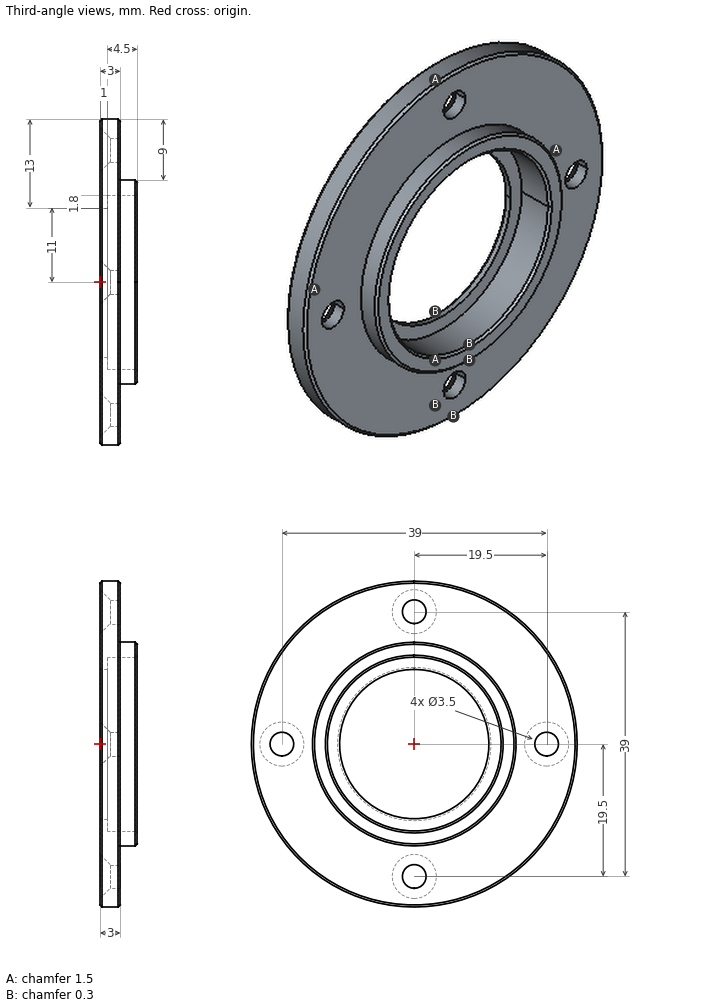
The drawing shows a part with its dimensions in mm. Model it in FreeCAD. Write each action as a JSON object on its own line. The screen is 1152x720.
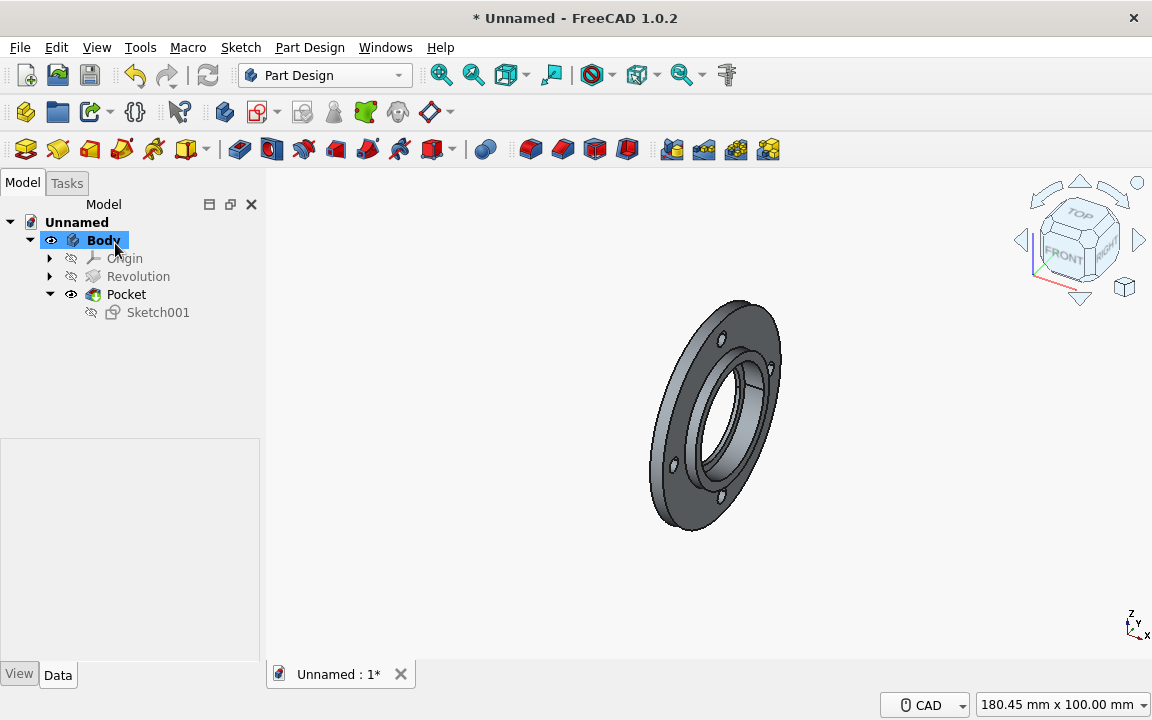
{"action": "key", "text": "0"}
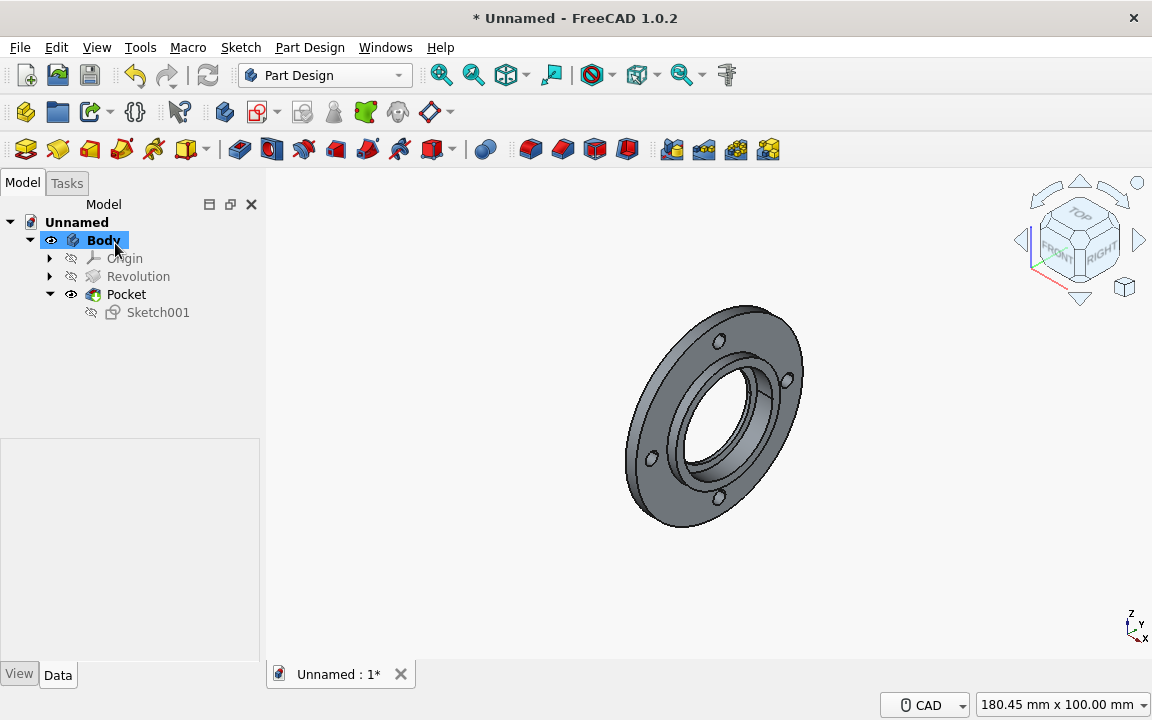
{"action": "key", "text": "2"}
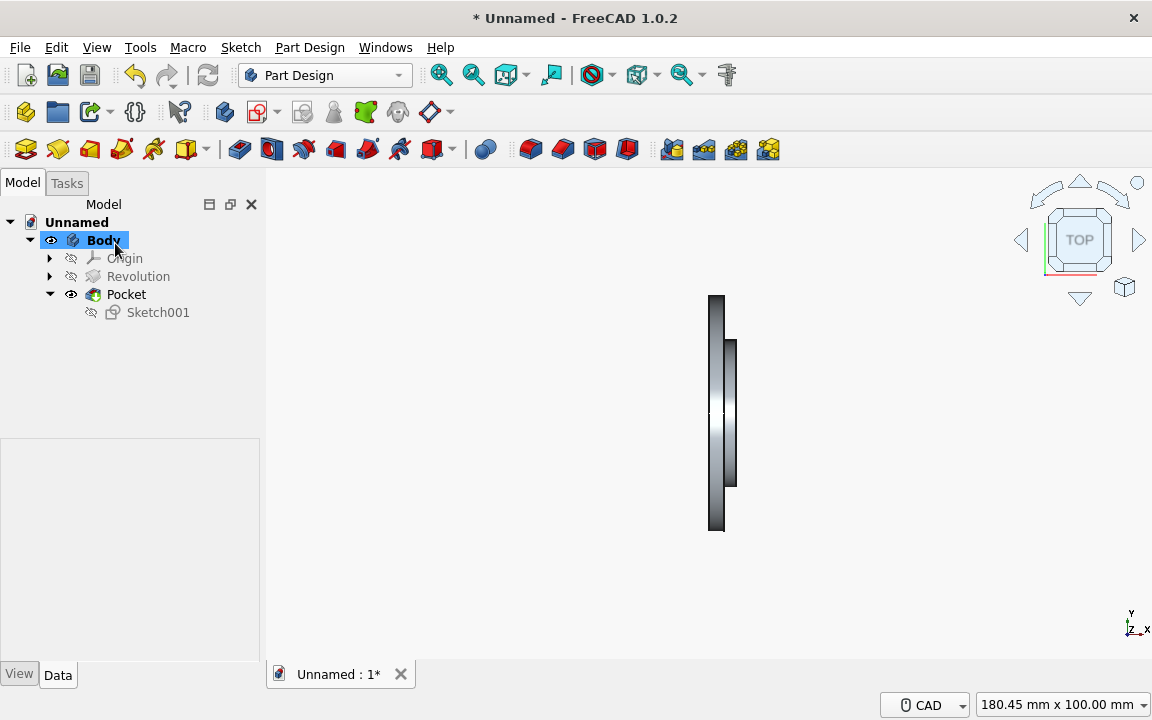
{"action": "key", "text": "1"}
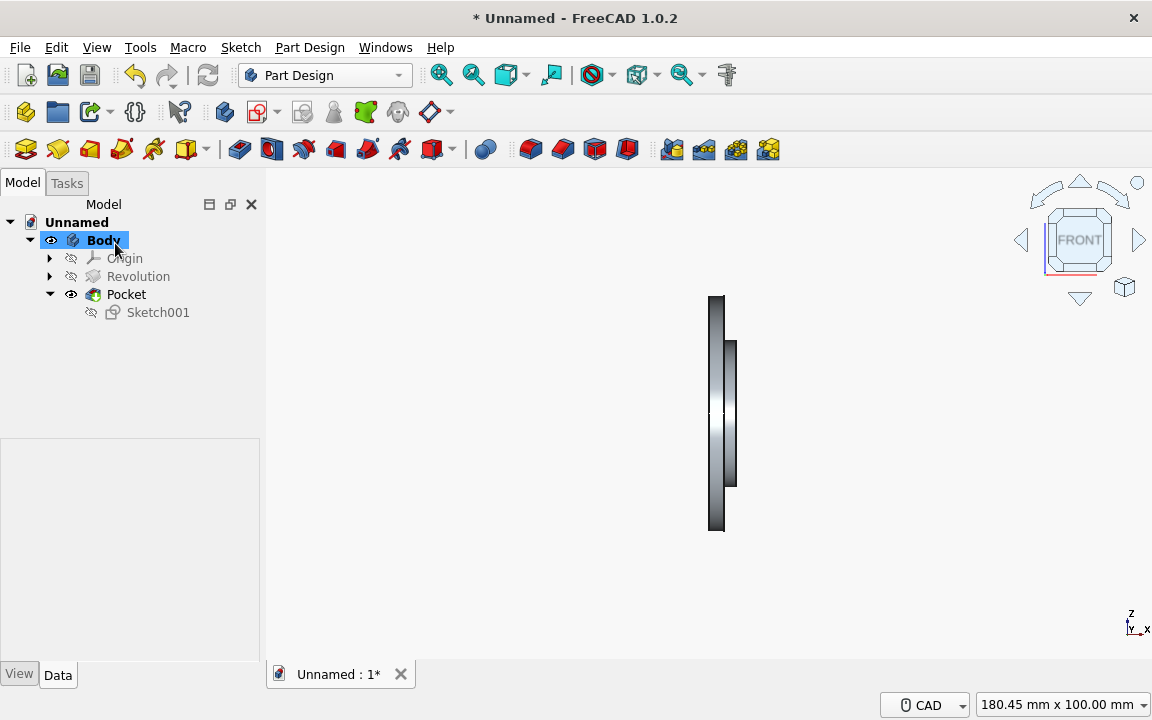
{"action": "key", "text": "3"}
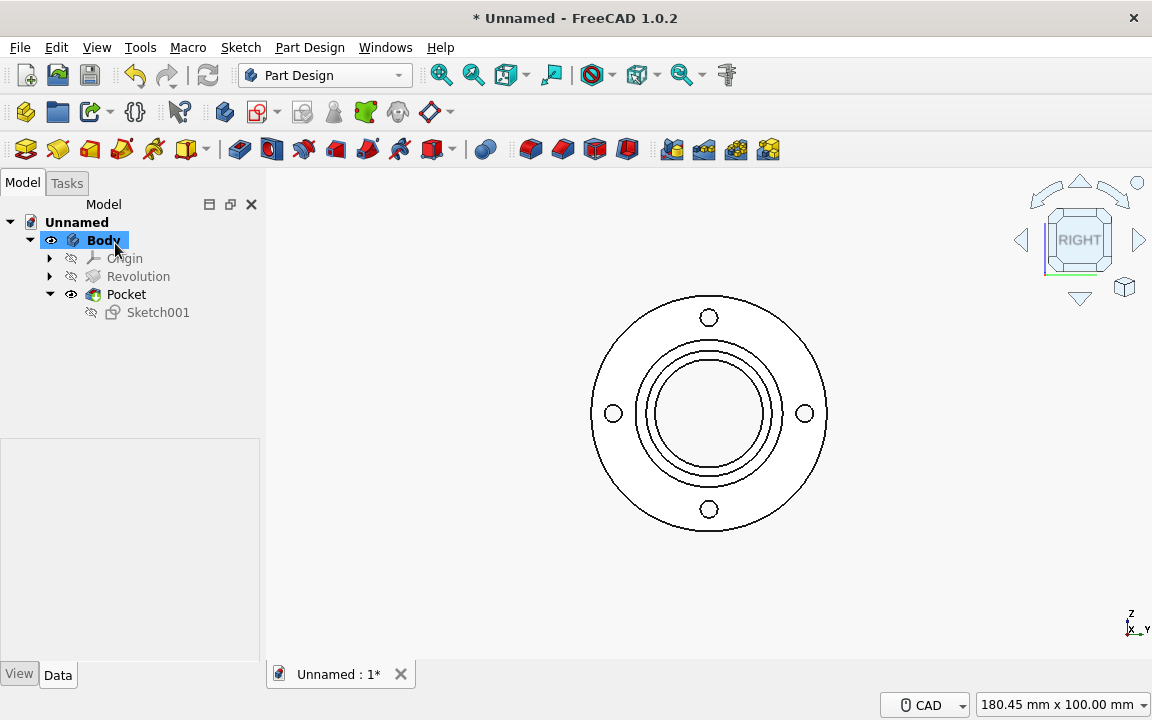
{"action": "key", "text": "5"}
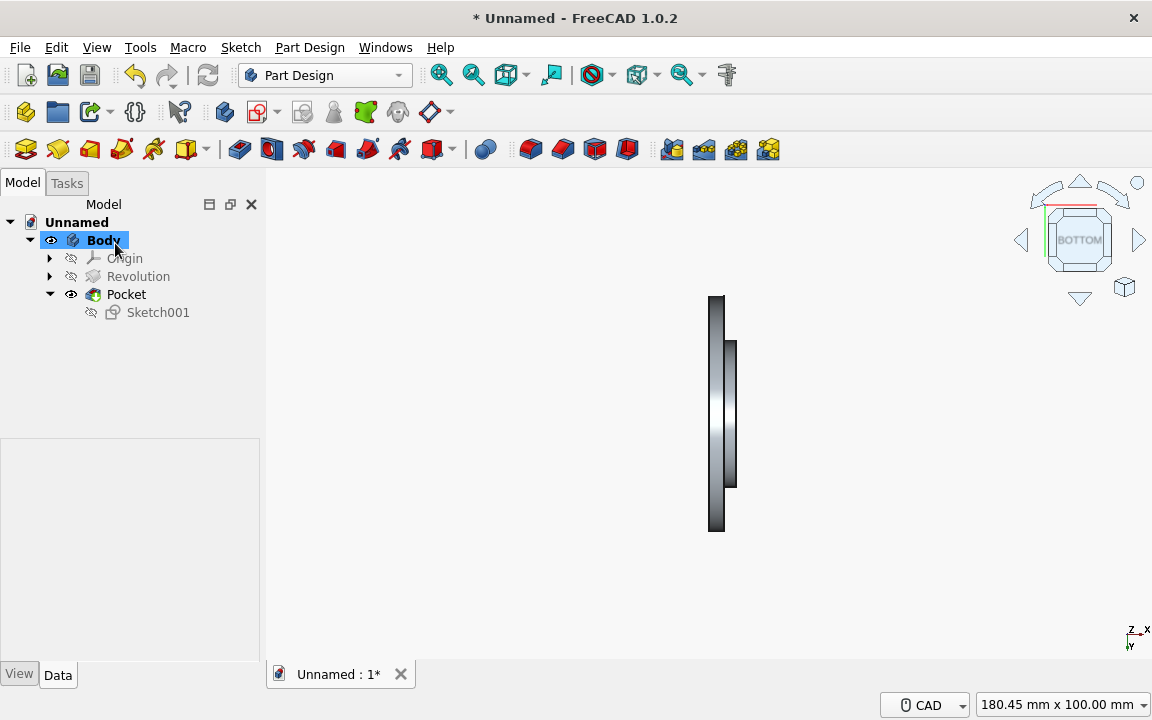
{"action": "key", "text": "4"}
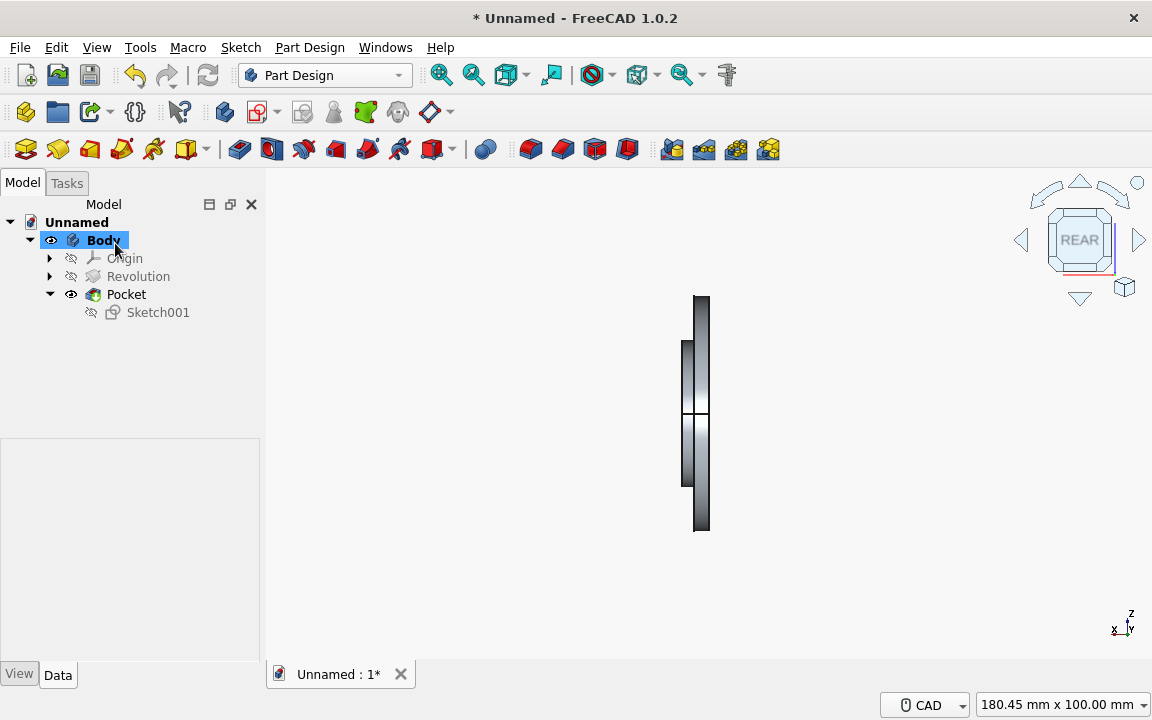
{"action": "key", "text": "6"}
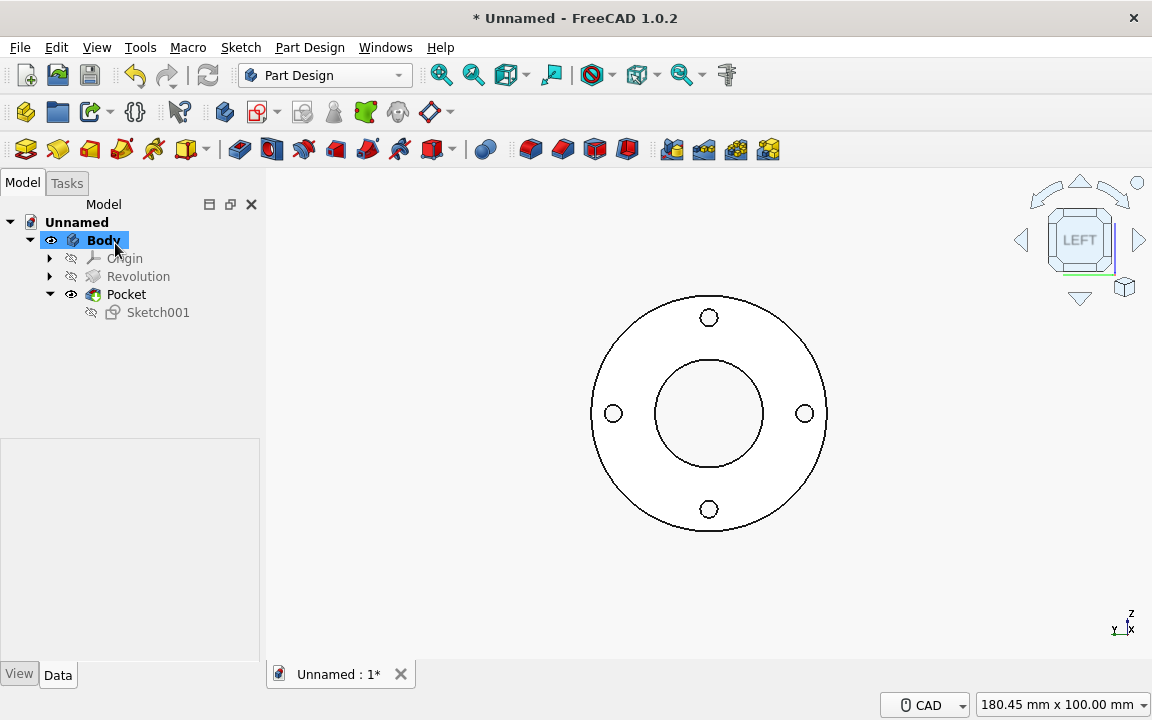
{"action": "left_click", "coordinate": [622, 412]}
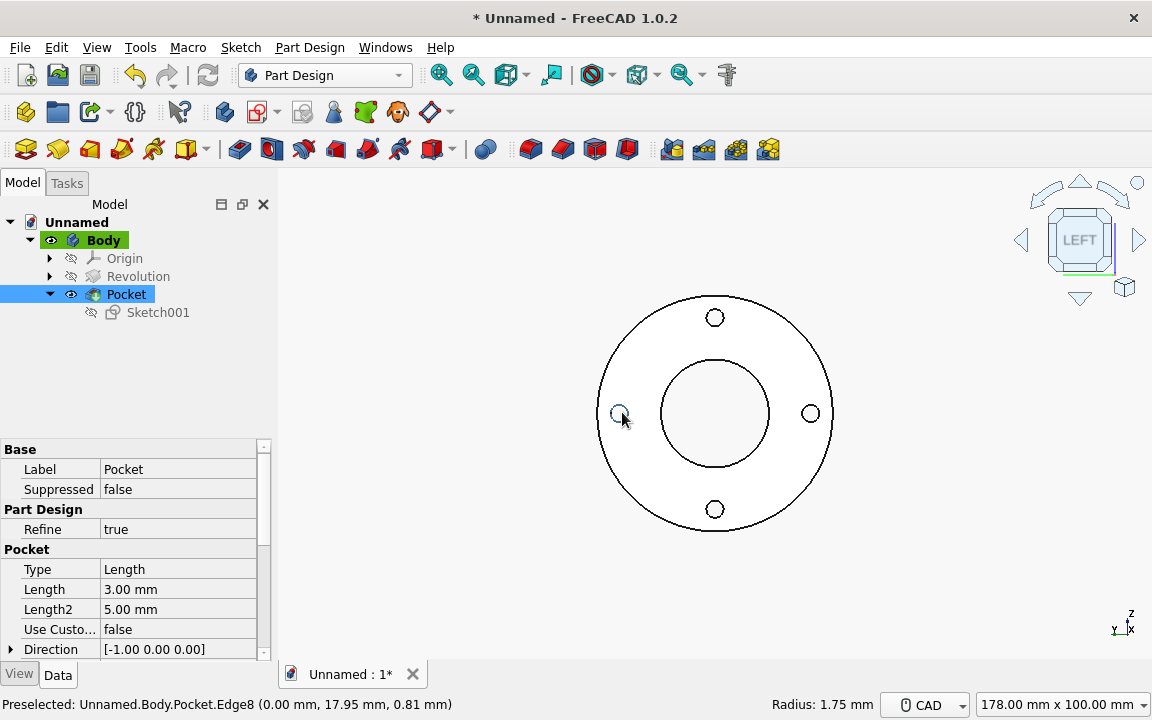
{"action": "left_click", "coordinate": [722, 503], "text": "ctrl"}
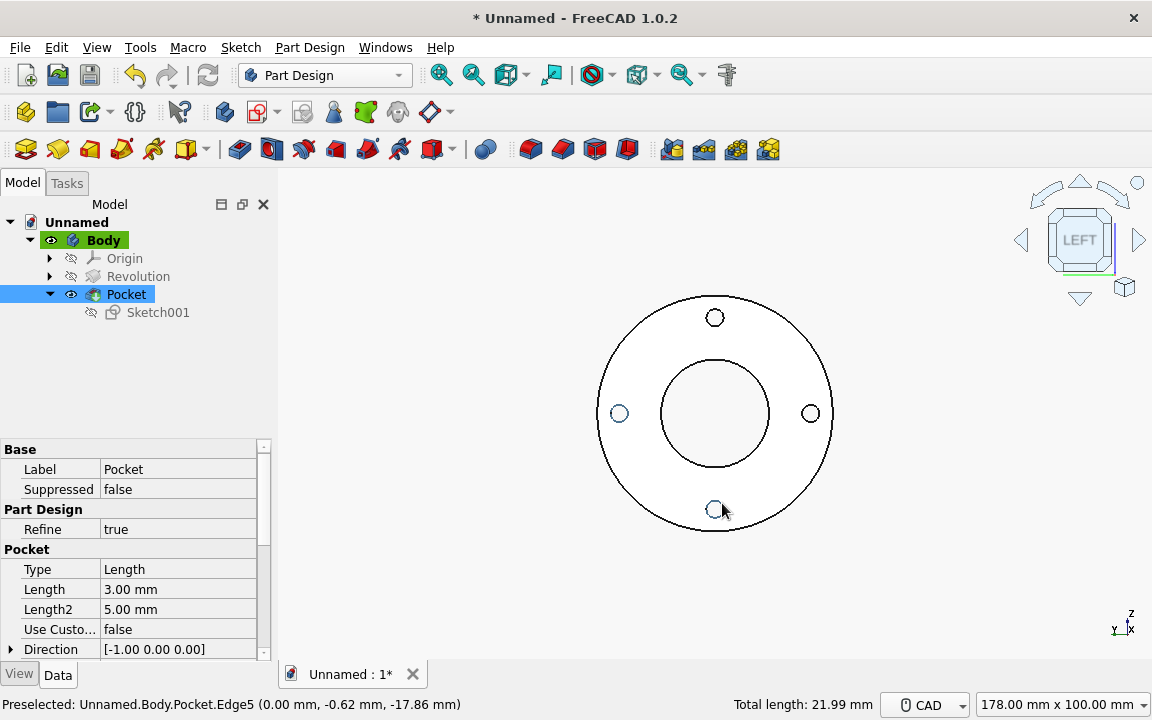
{"action": "left_click", "coordinate": [813, 404], "text": "ctrl"}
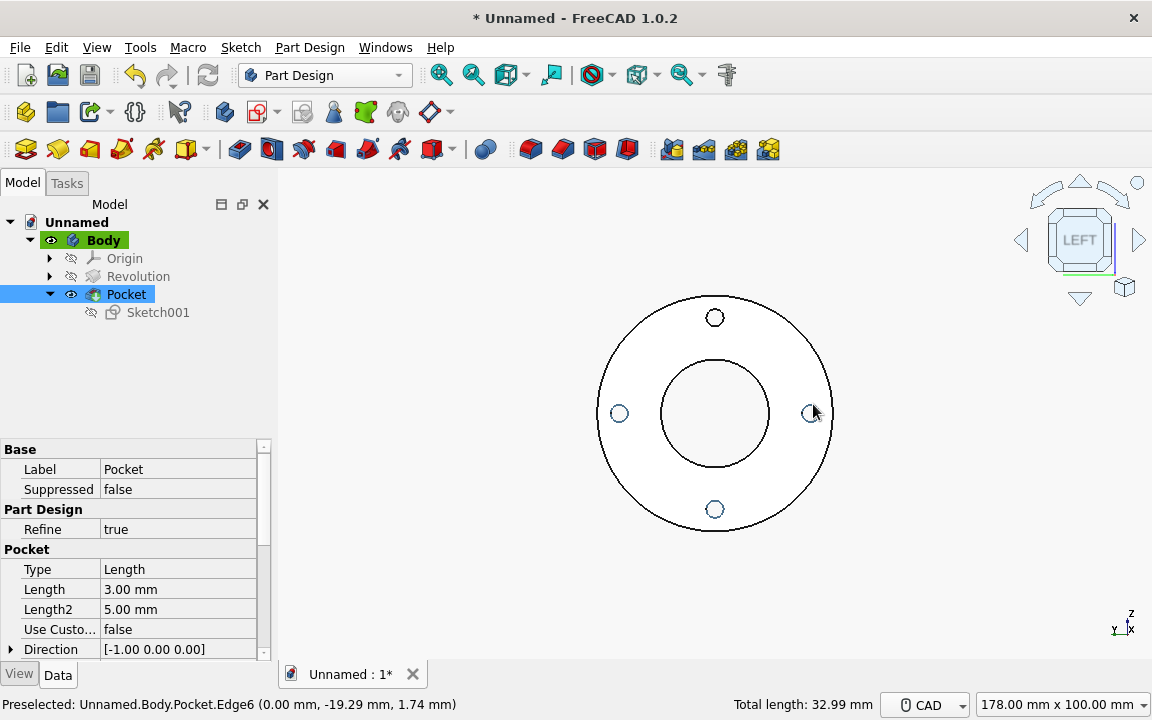
{"action": "left_click", "coordinate": [722, 322], "text": "ctrl"}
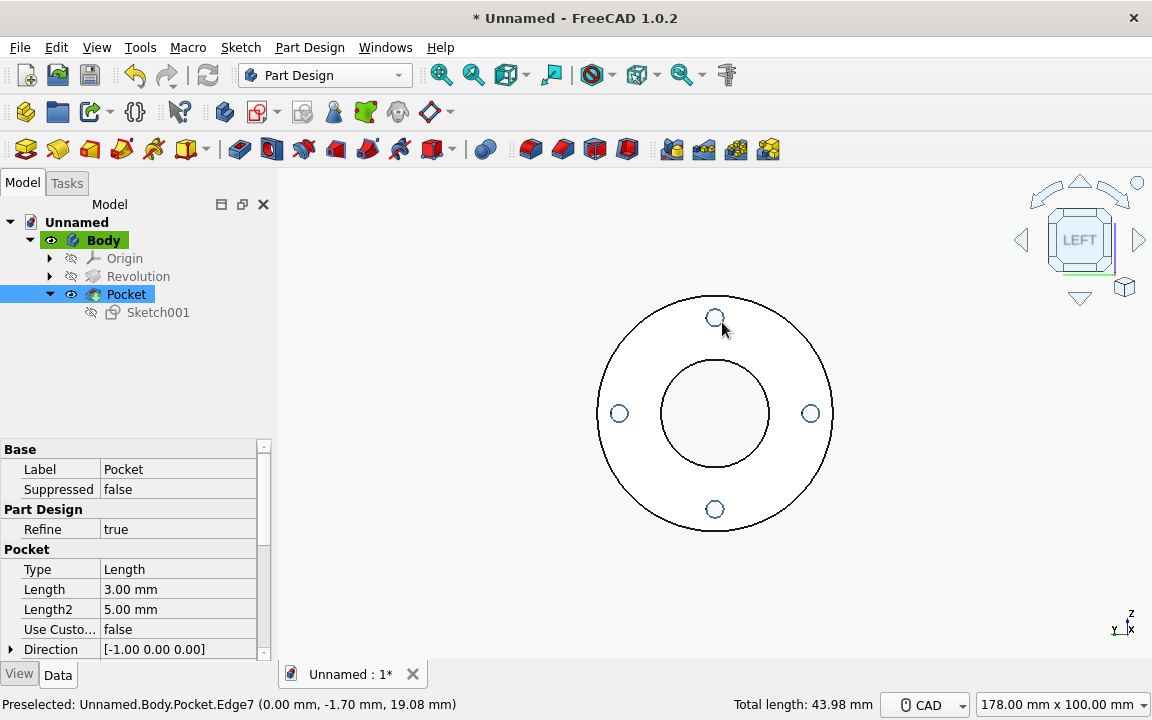
{"action": "left_click", "coordinate": [564, 150]}